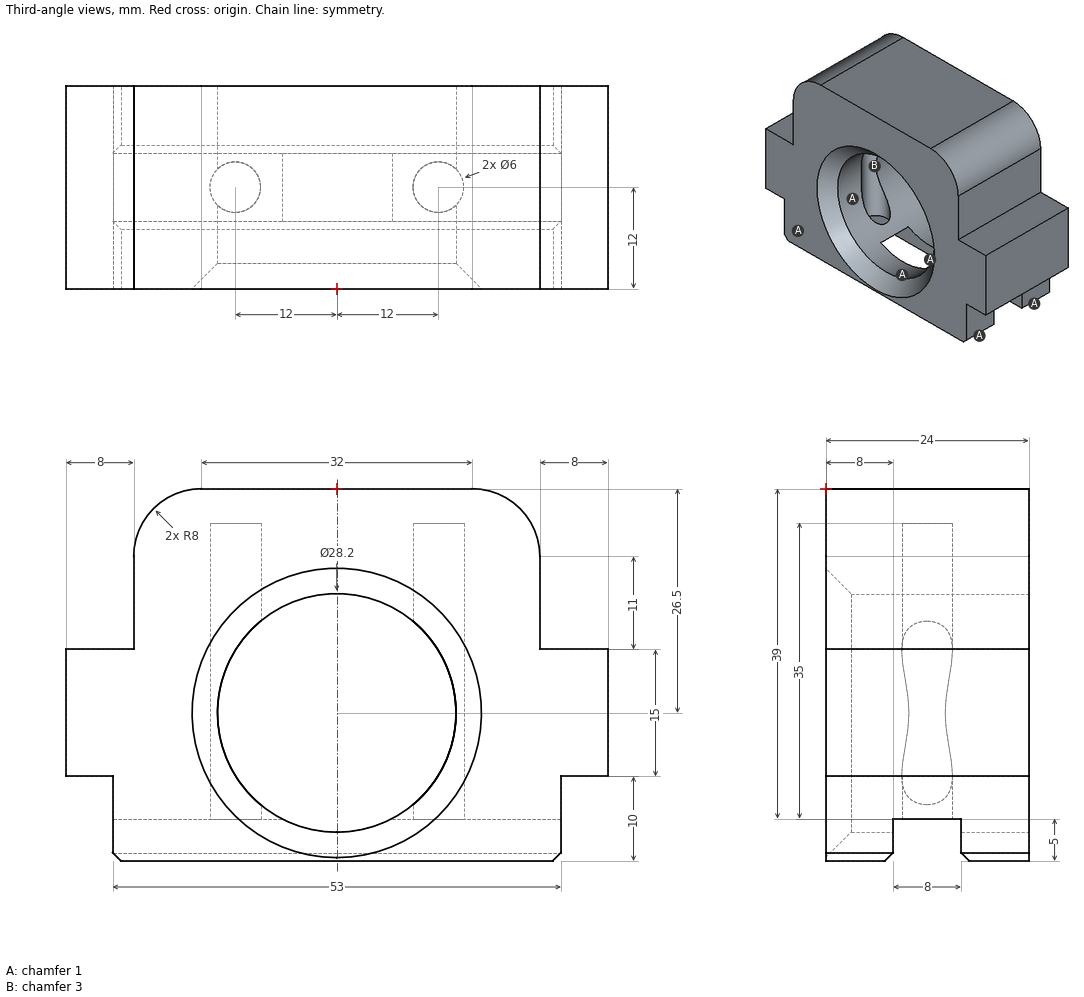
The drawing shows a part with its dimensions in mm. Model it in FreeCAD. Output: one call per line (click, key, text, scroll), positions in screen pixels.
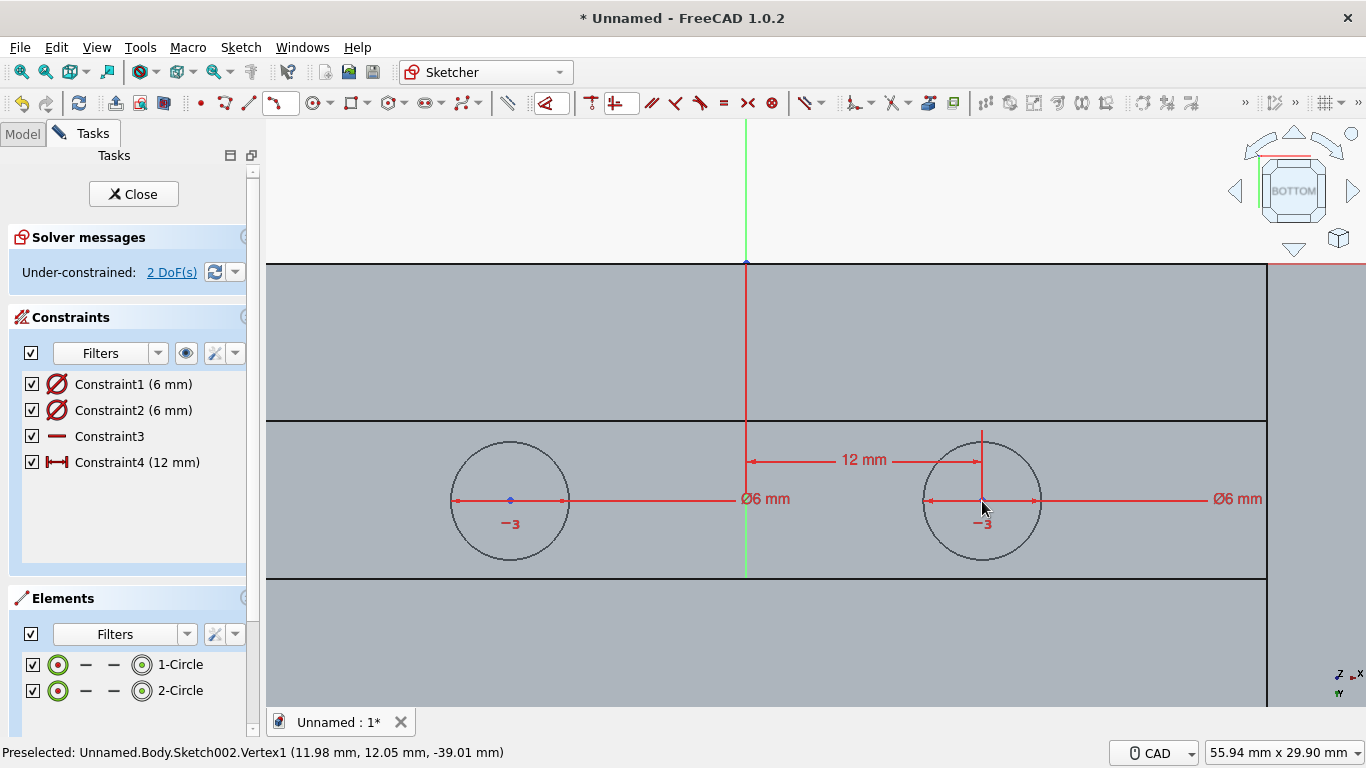
click(982, 501)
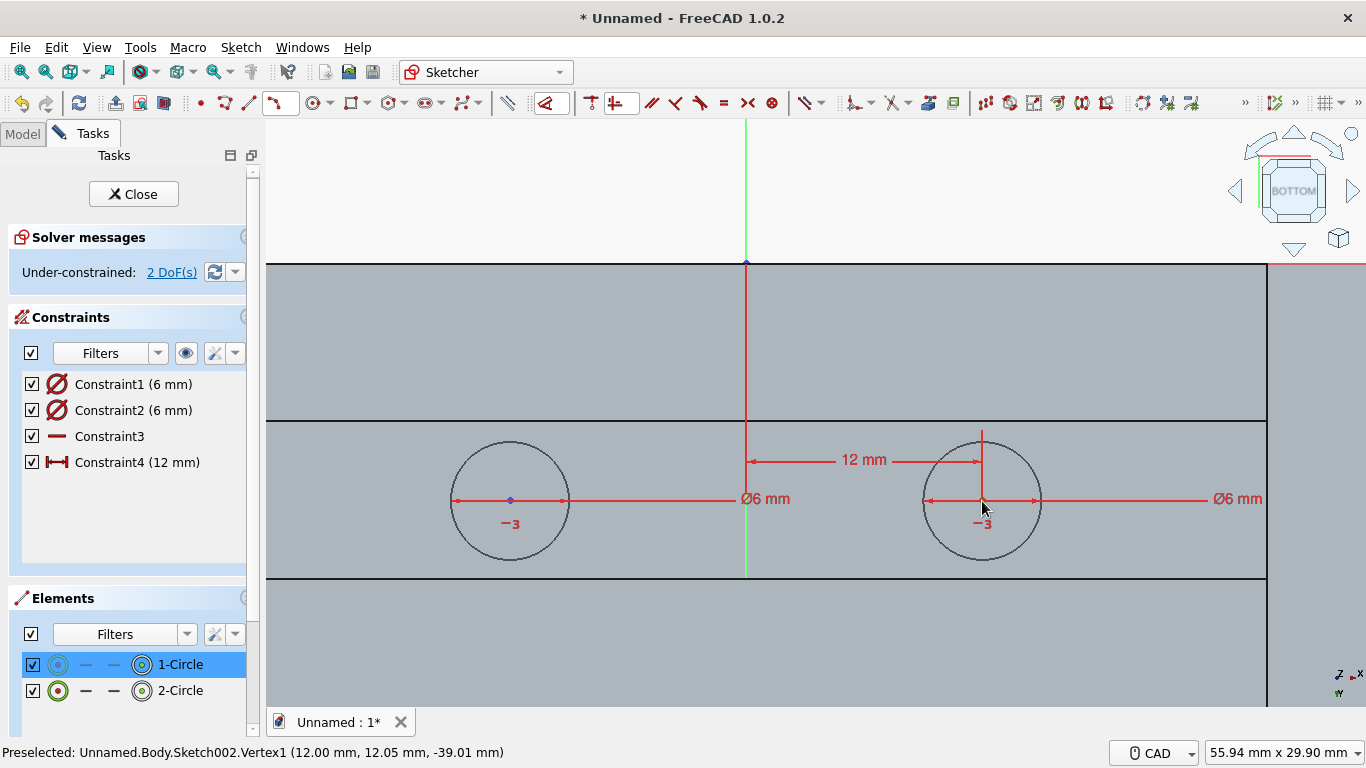
key(i)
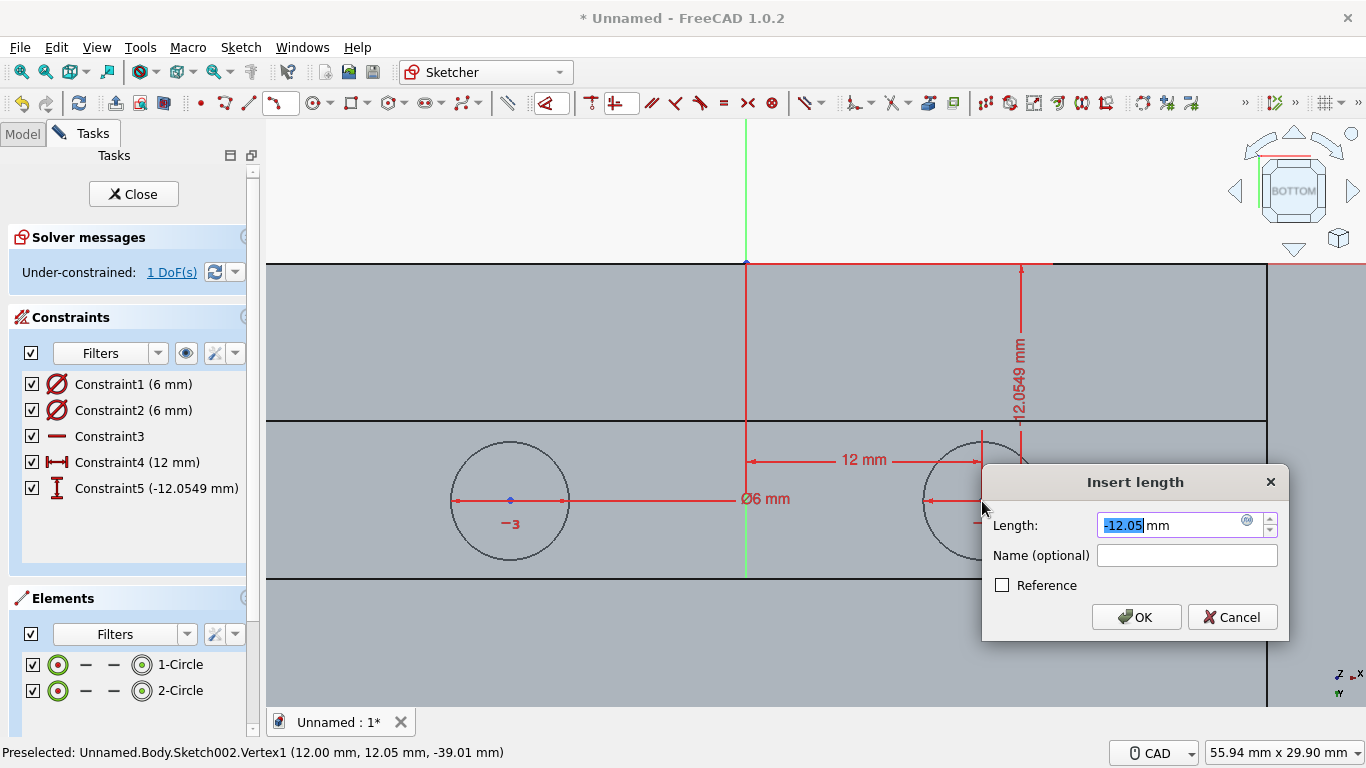
text(-12)
key(Return)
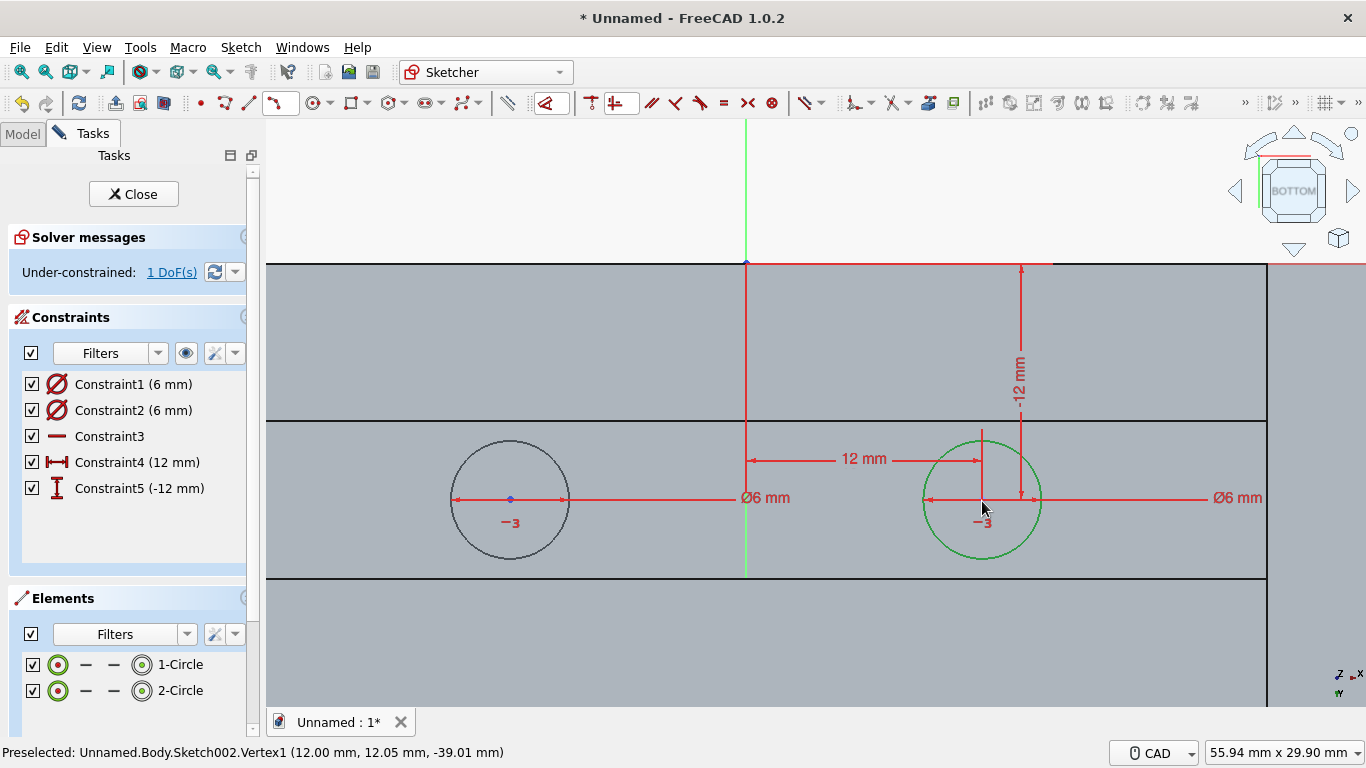
click(510, 500)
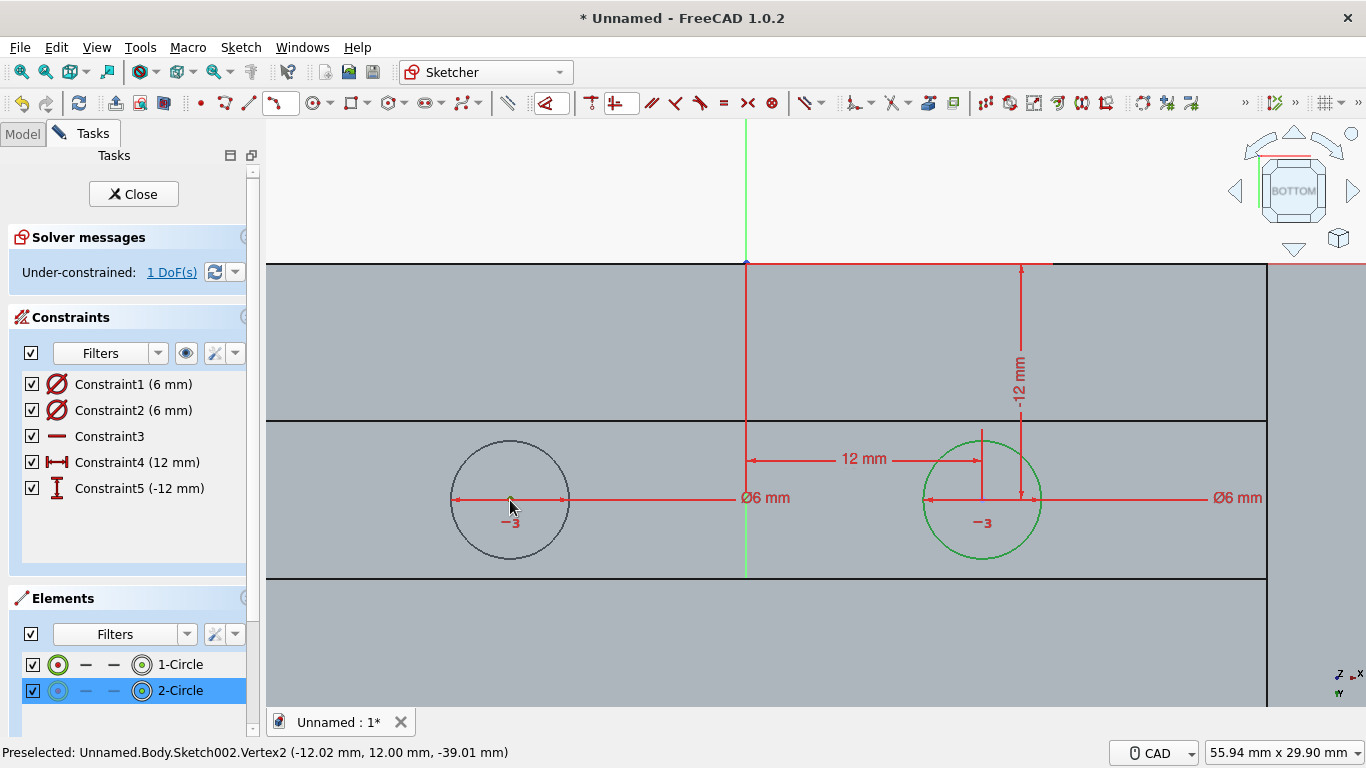
click(564, 104)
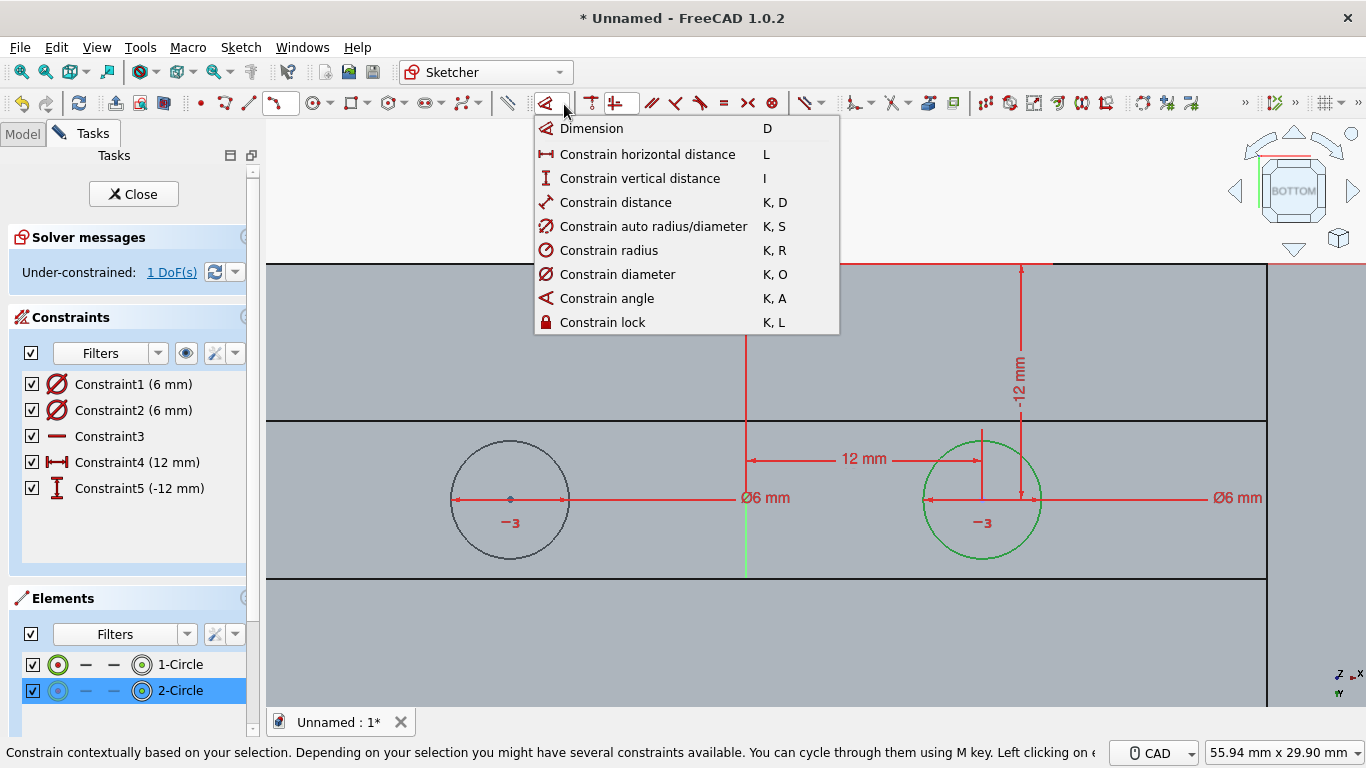
click(687, 154)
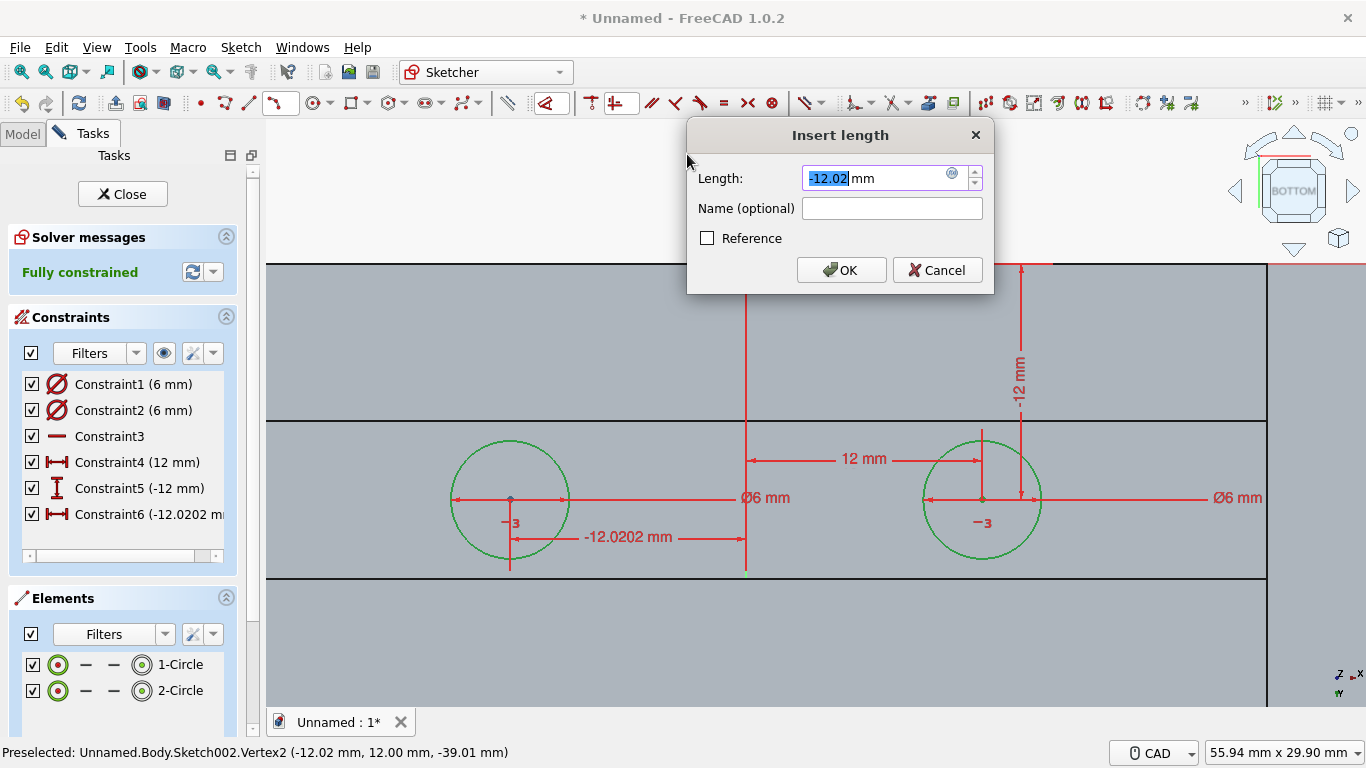
text(-12)
key(Return)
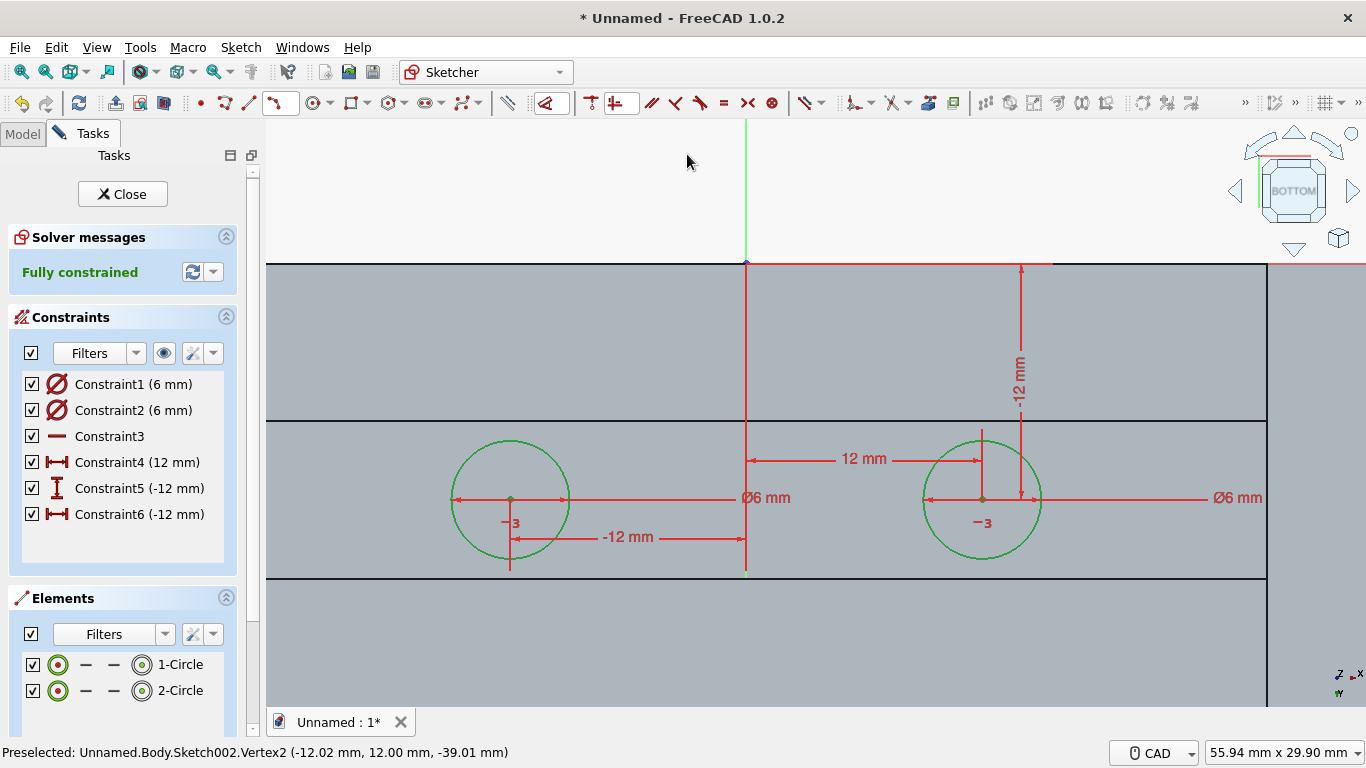
click(123, 194)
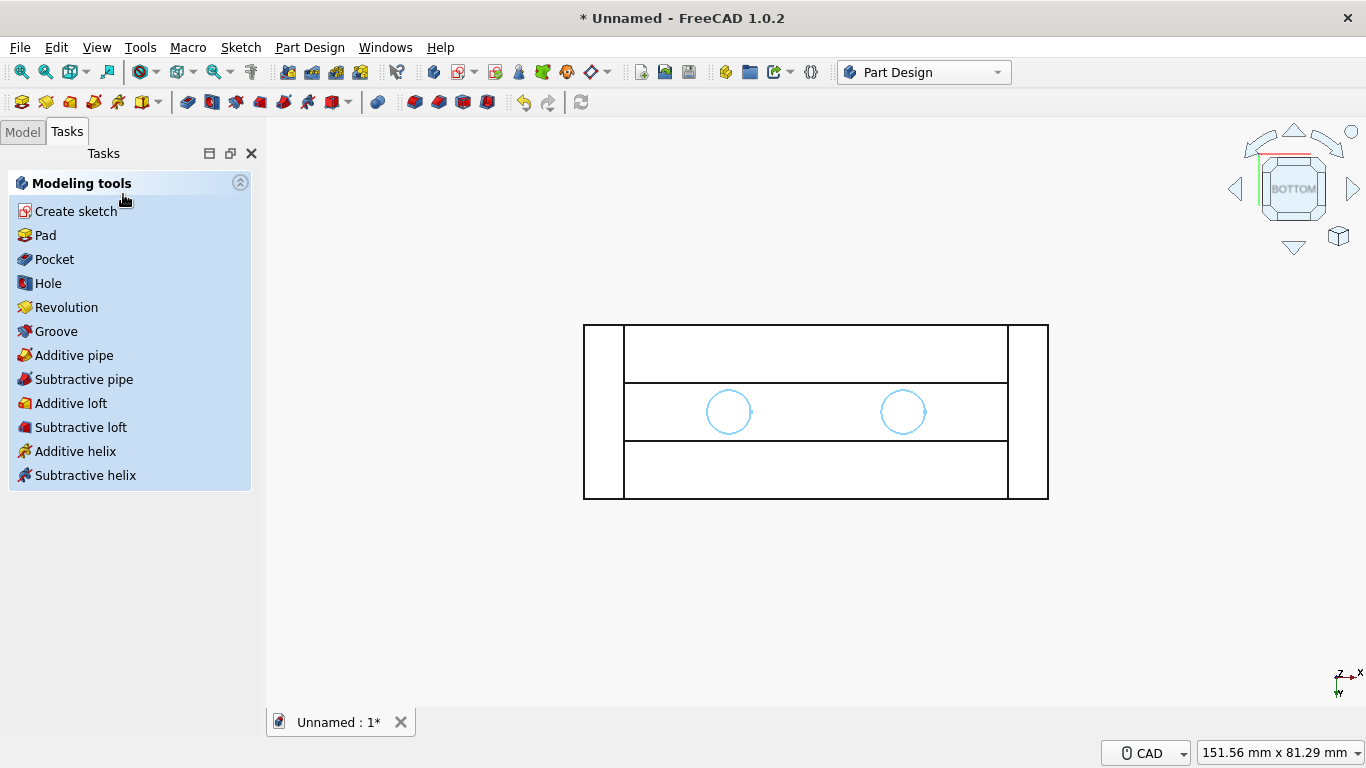
click(188, 102)